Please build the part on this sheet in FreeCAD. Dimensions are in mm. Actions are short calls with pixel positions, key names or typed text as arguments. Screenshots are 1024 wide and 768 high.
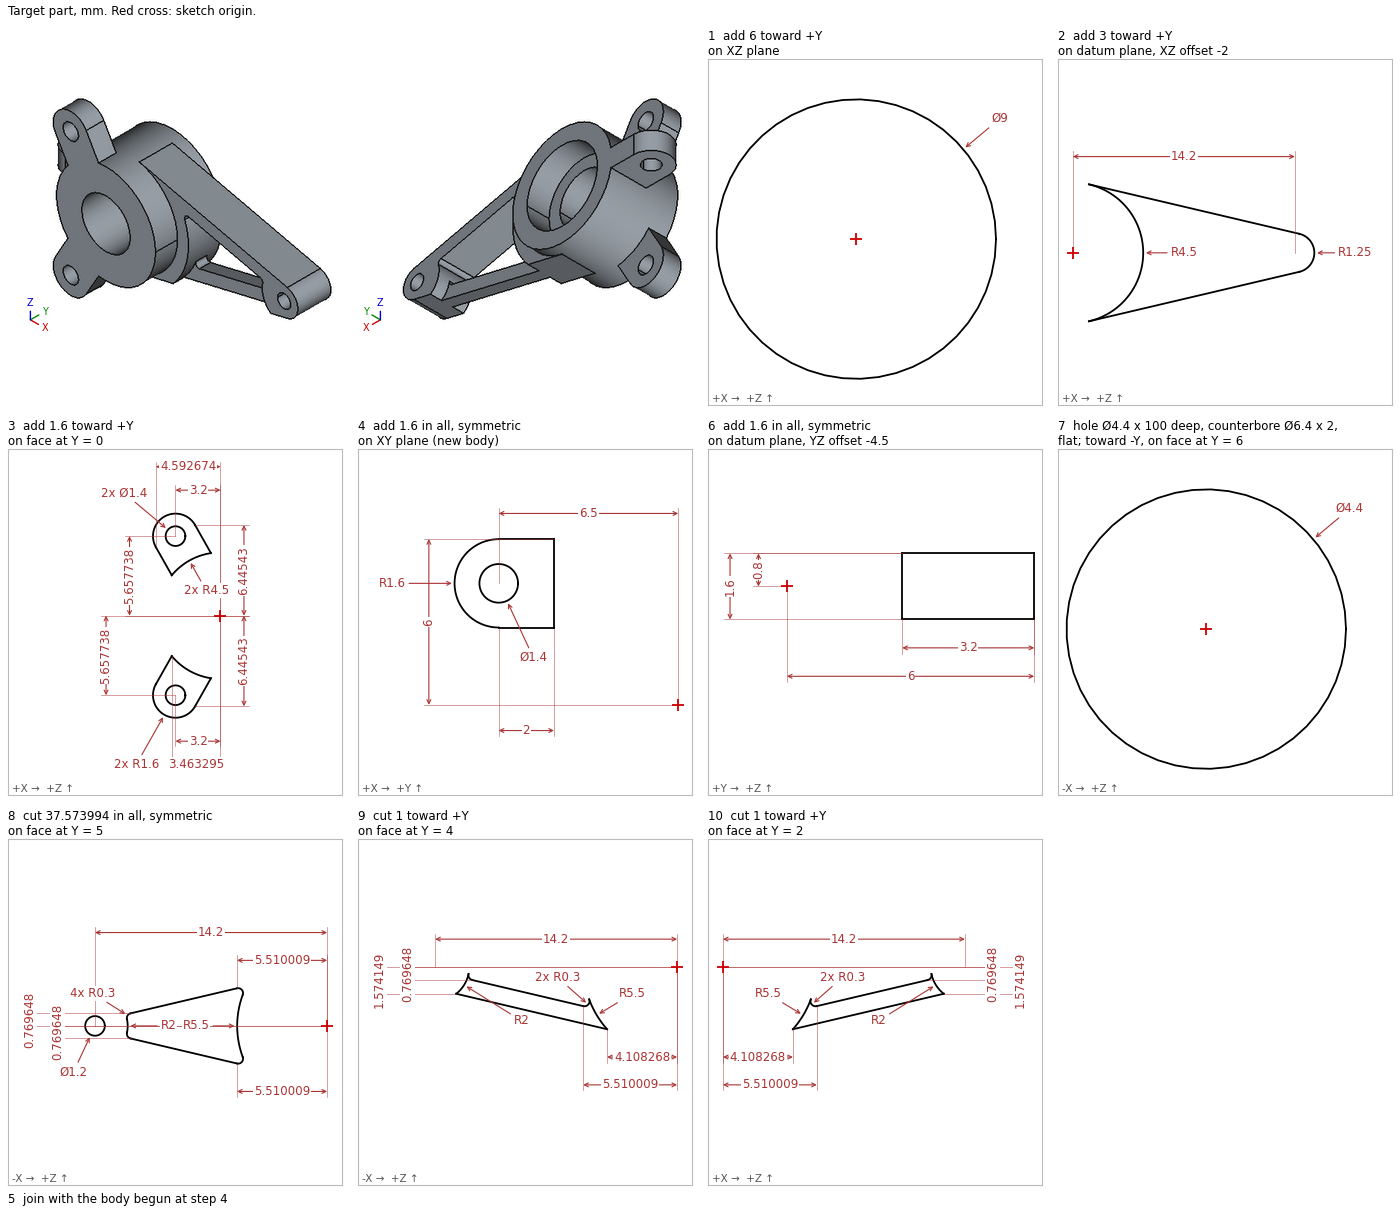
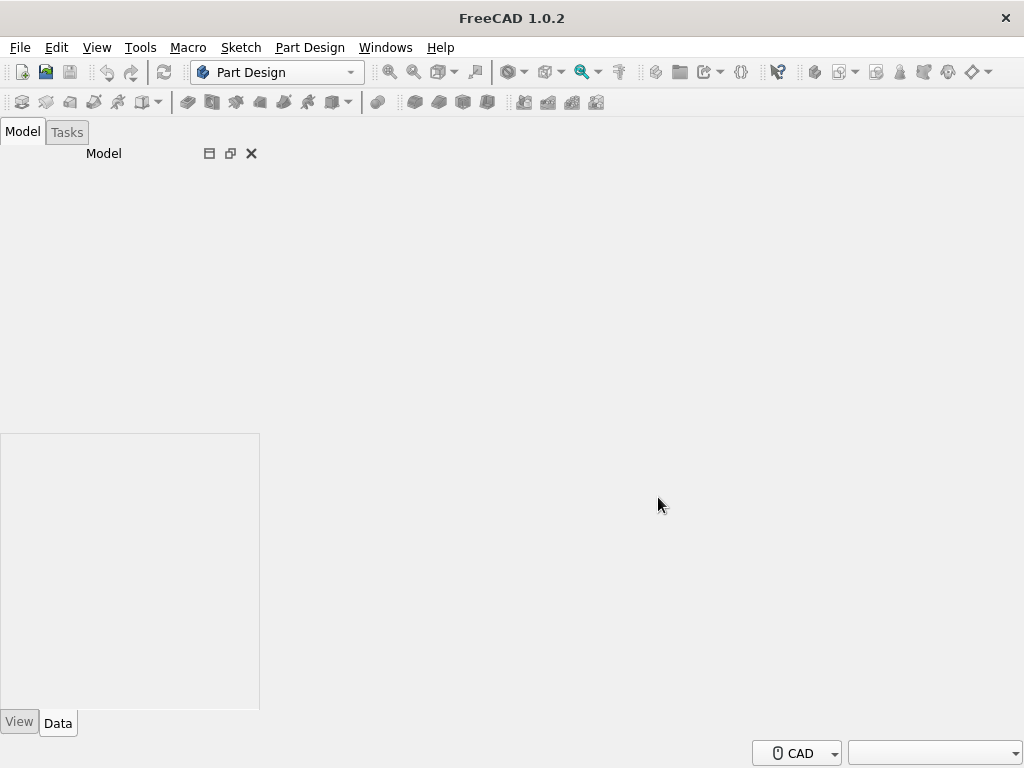
click(22, 72)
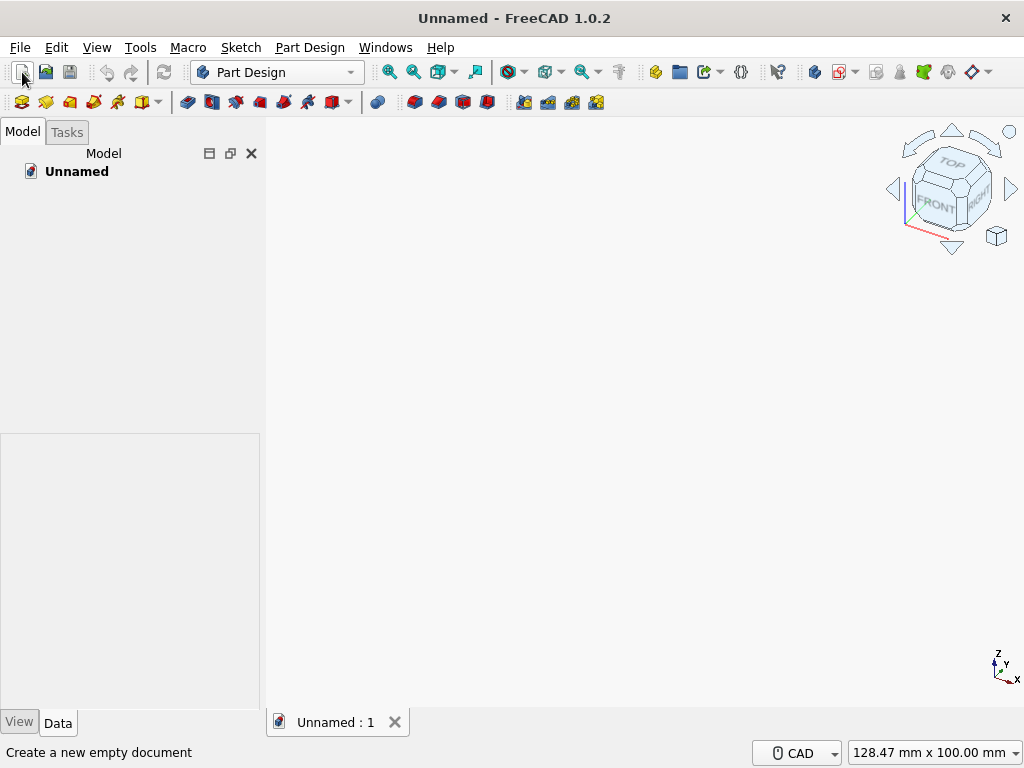
click(840, 72)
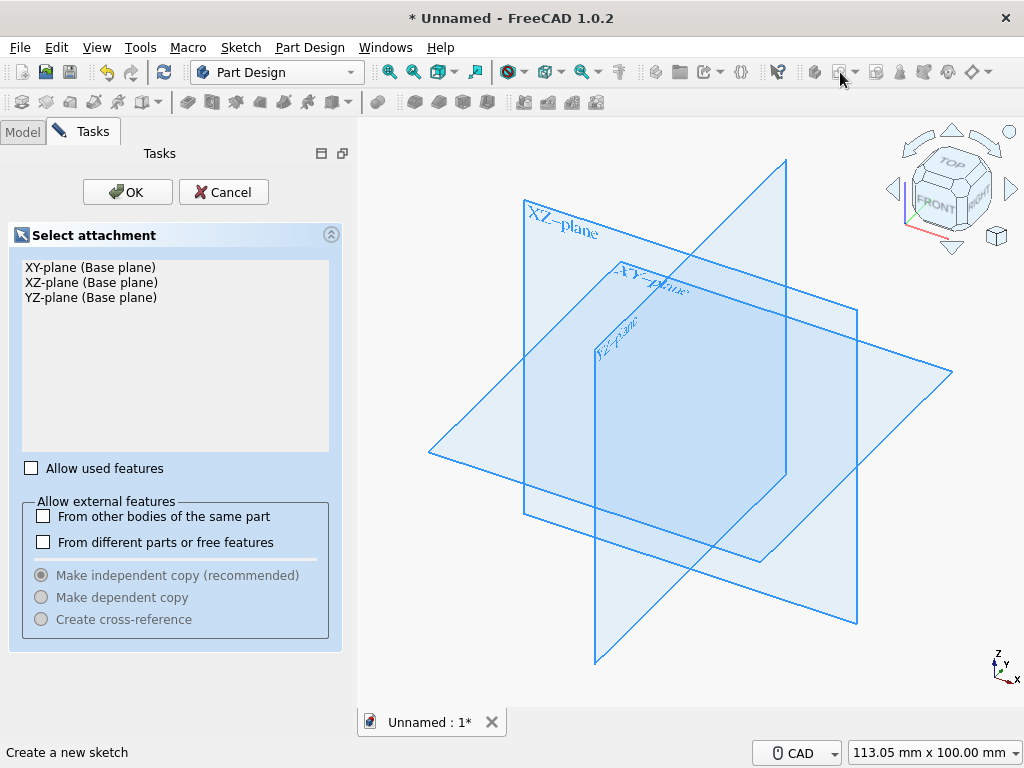
click(82, 282)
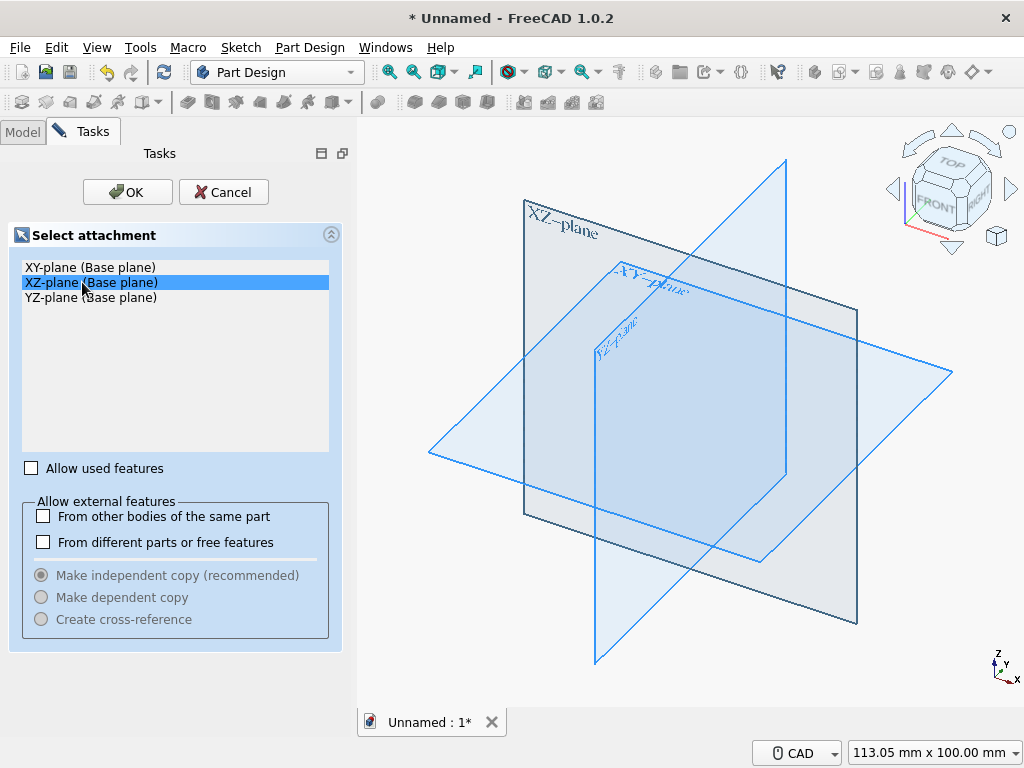
click(128, 192)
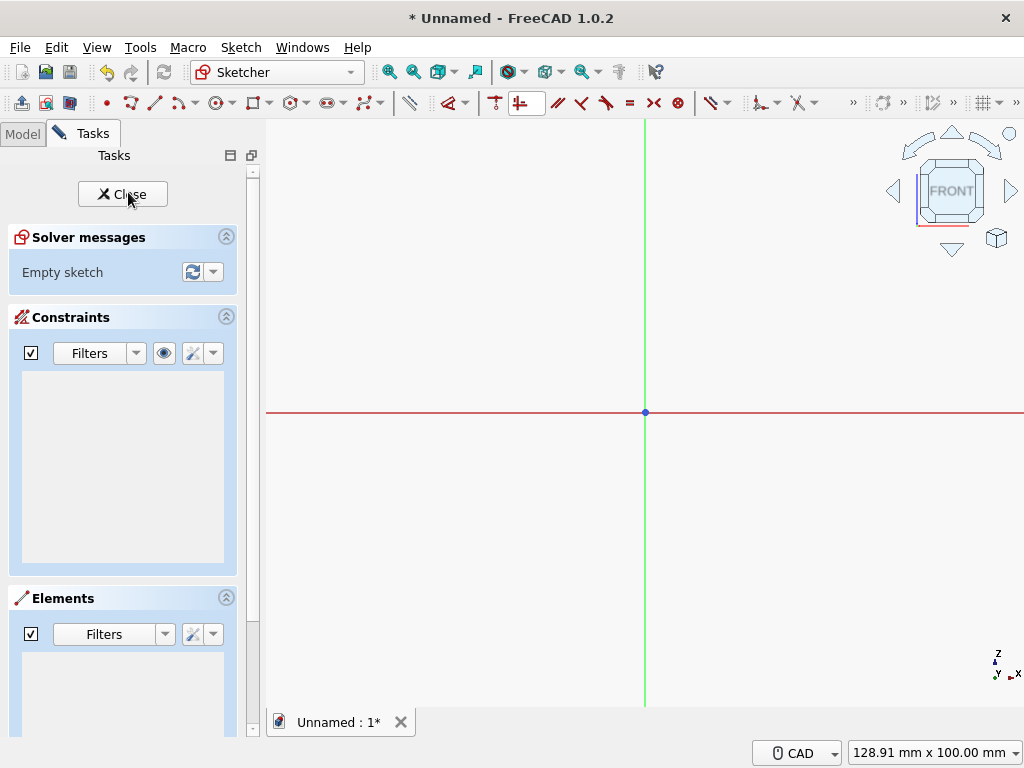
scroll(656, 413, up, 10)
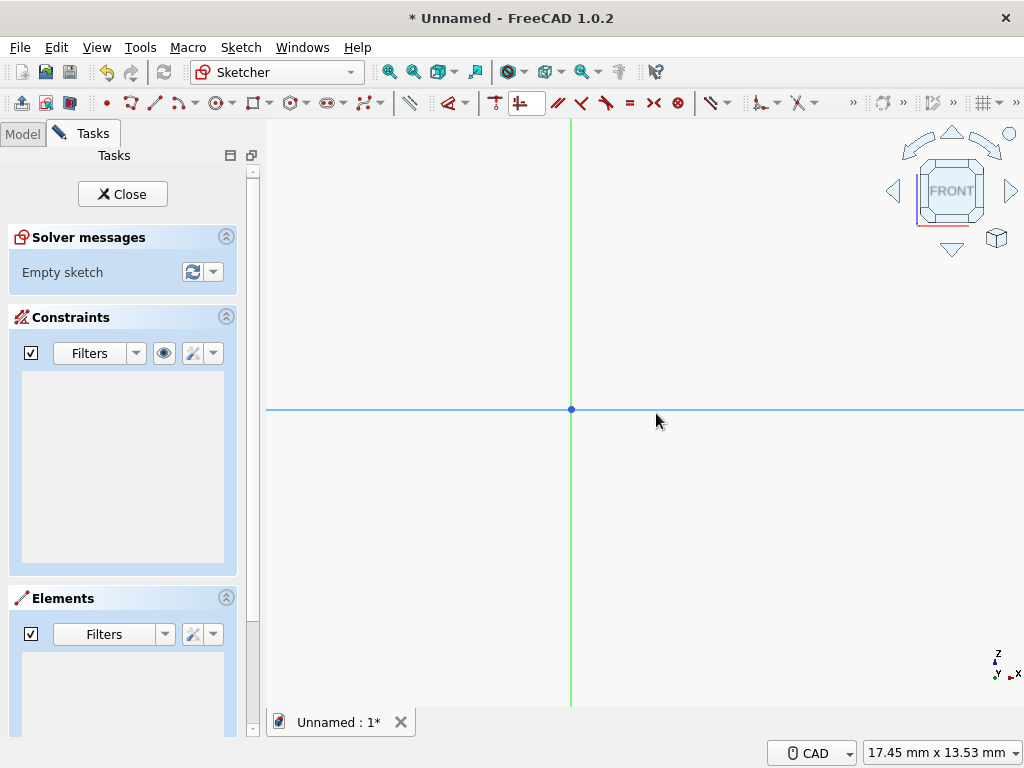
key(g)
key(c)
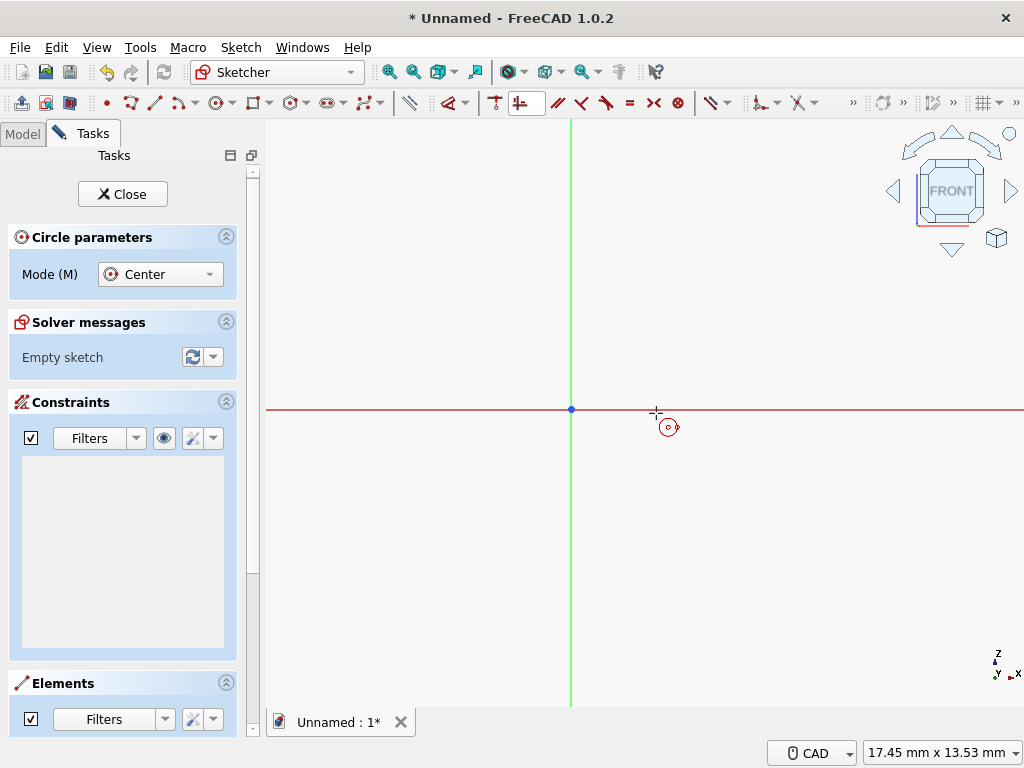
click(571, 410)
click(710, 272)
key(Escape)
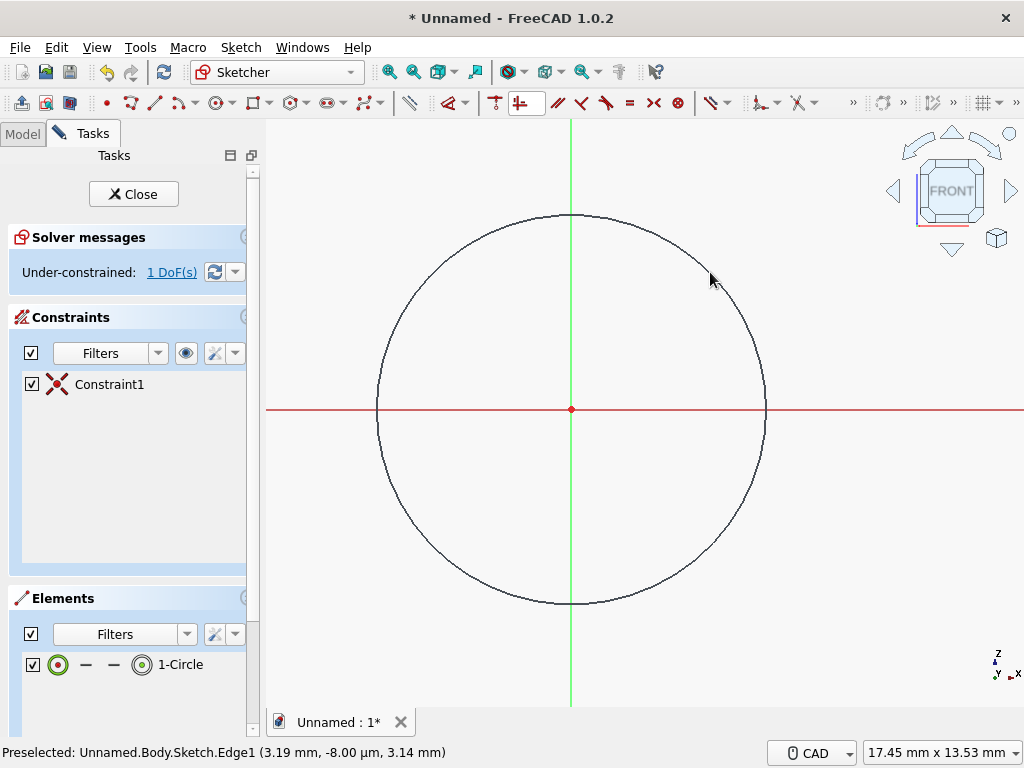
key(d)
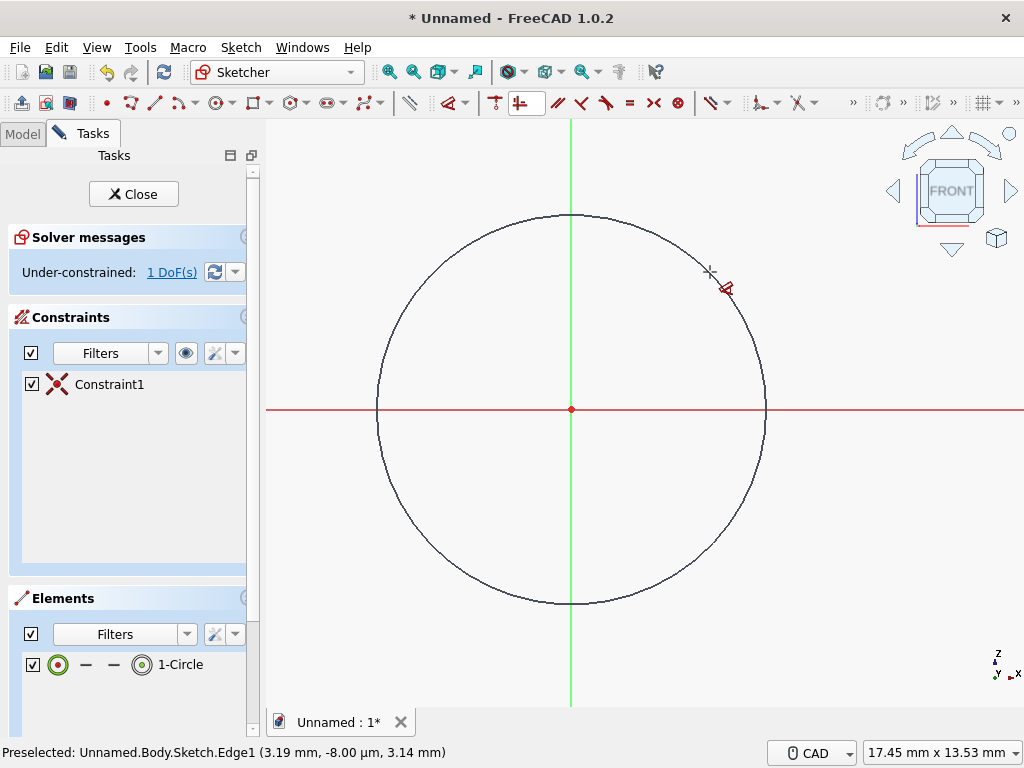
click(709, 272)
click(732, 249)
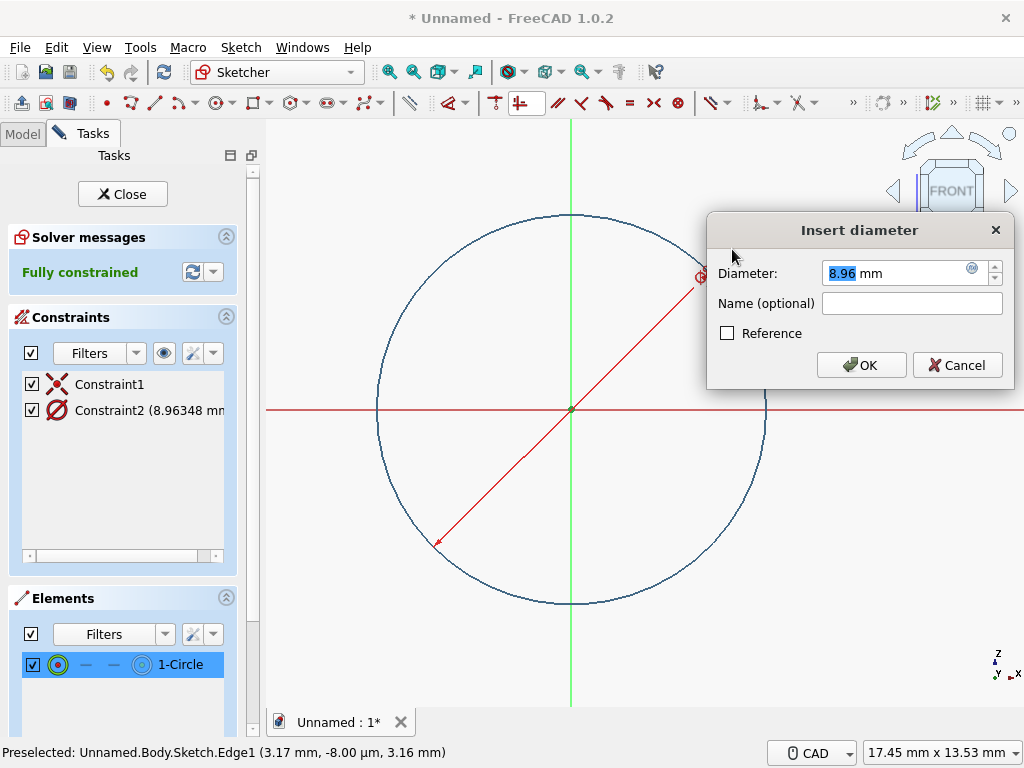
text(9)
key(Return)
key(Escape)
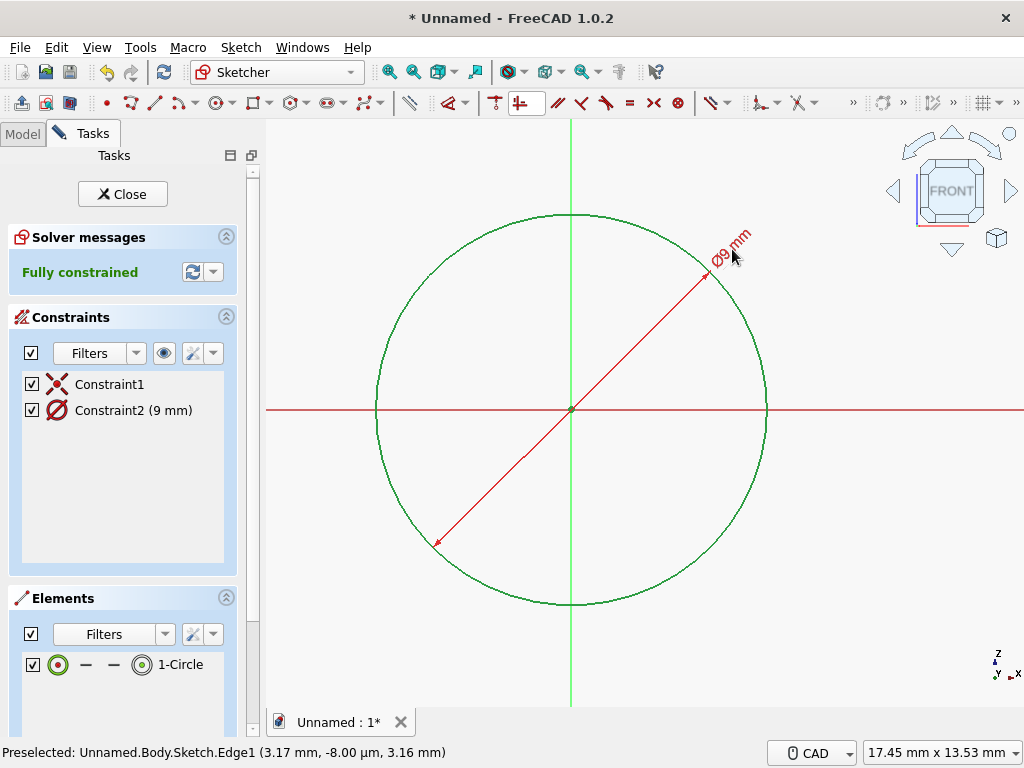
click(123, 194)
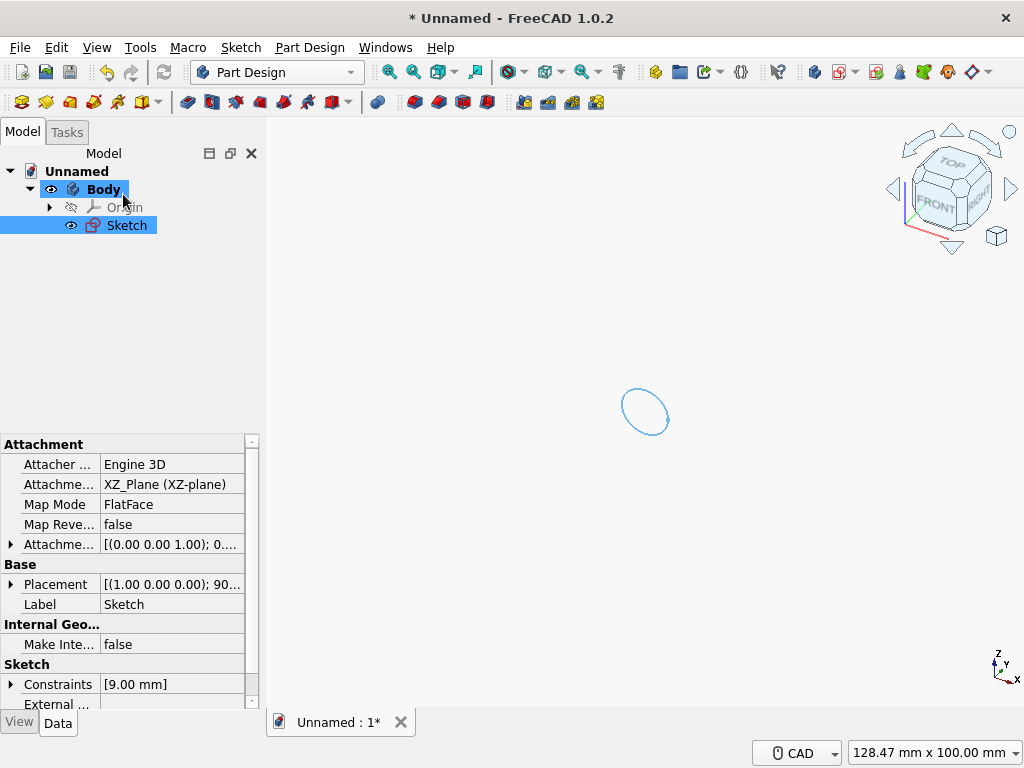
click(22, 102)